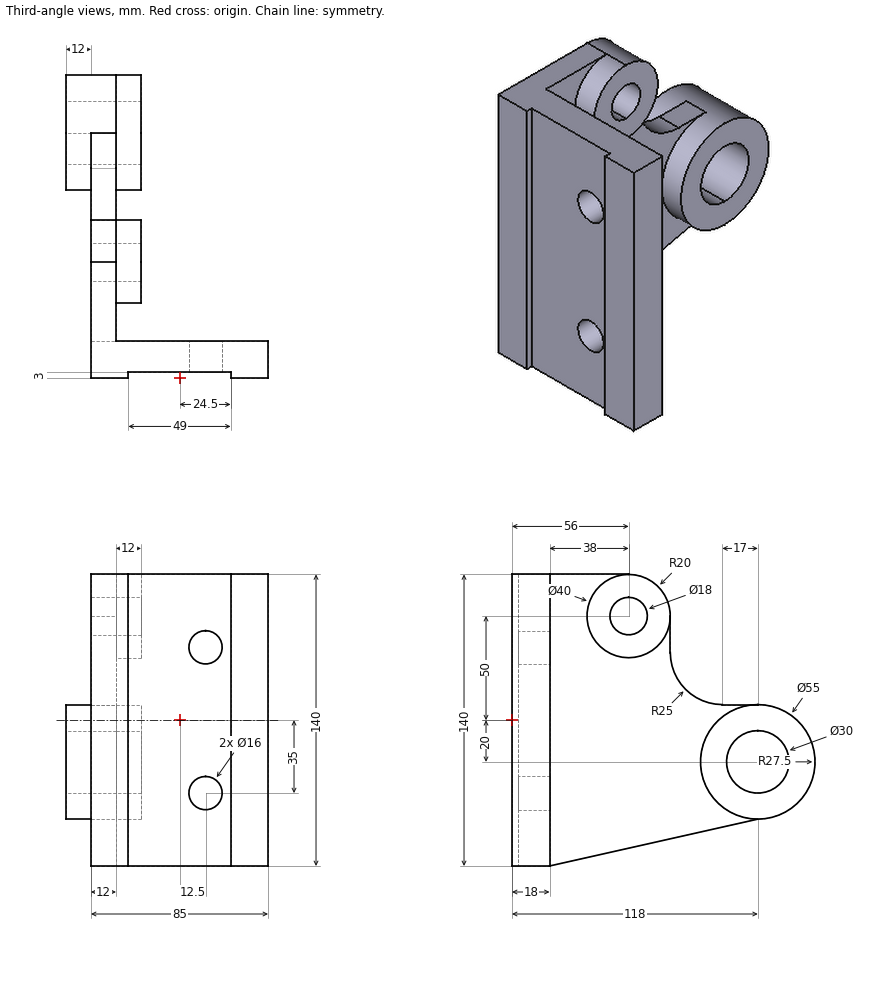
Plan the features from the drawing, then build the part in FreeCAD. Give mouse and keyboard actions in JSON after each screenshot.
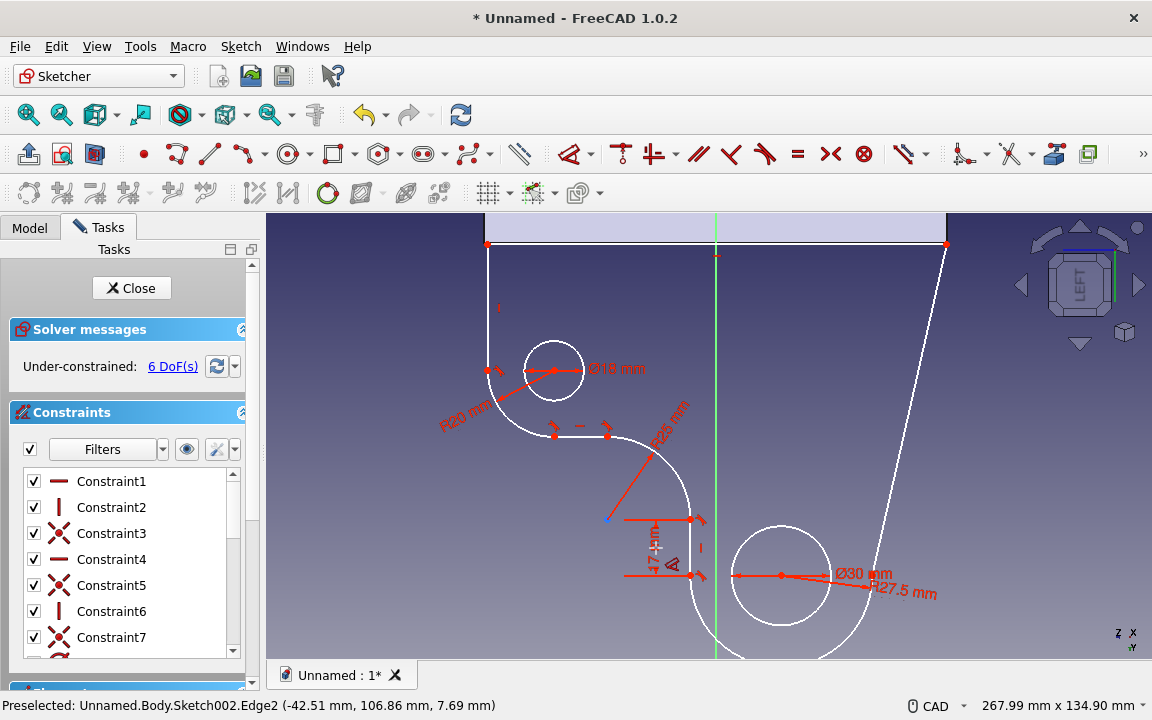
{"action": "left_click", "coordinate": [488, 282]}
{"action": "left_click", "coordinate": [454, 308]}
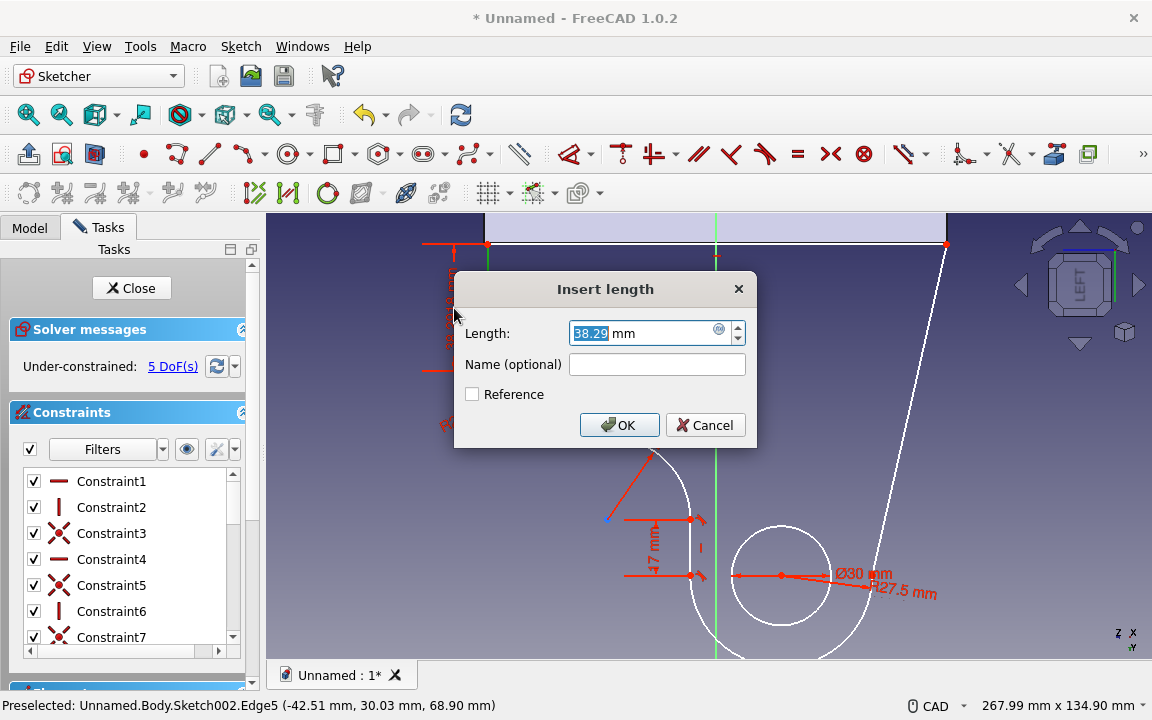
{"action": "type", "text": "38"}
{"action": "key", "text": "Return"}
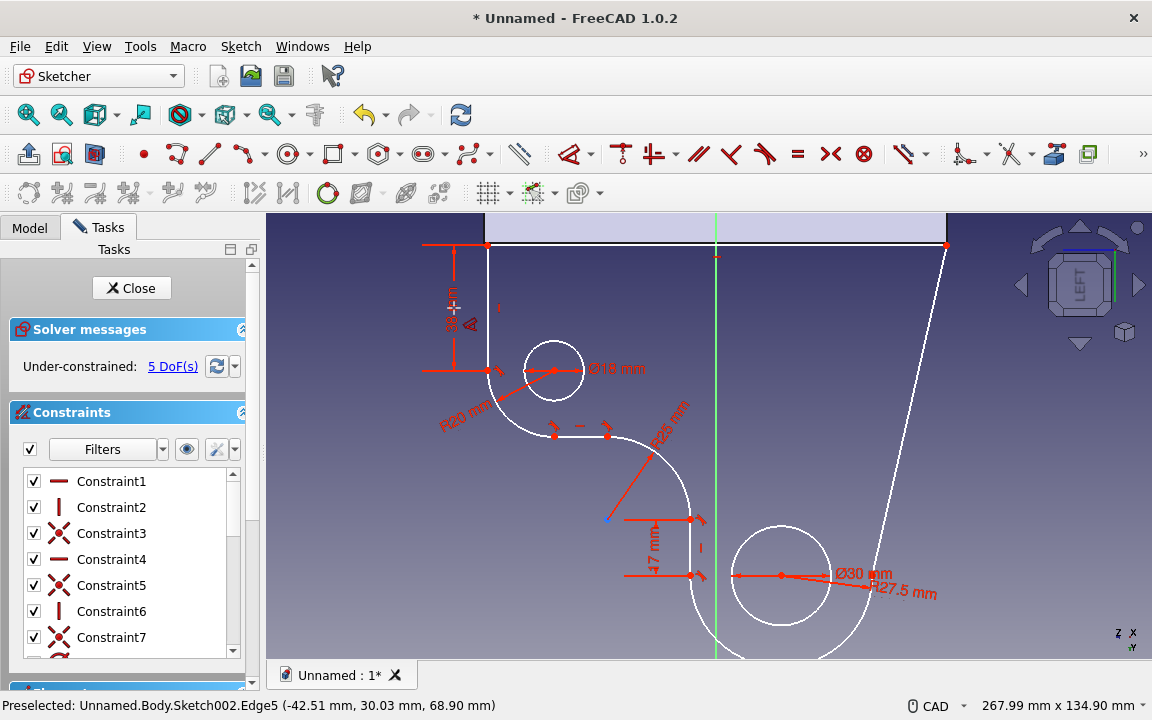
{"action": "left_click", "coordinate": [554, 371]}
{"action": "left_click", "coordinate": [635, 405]}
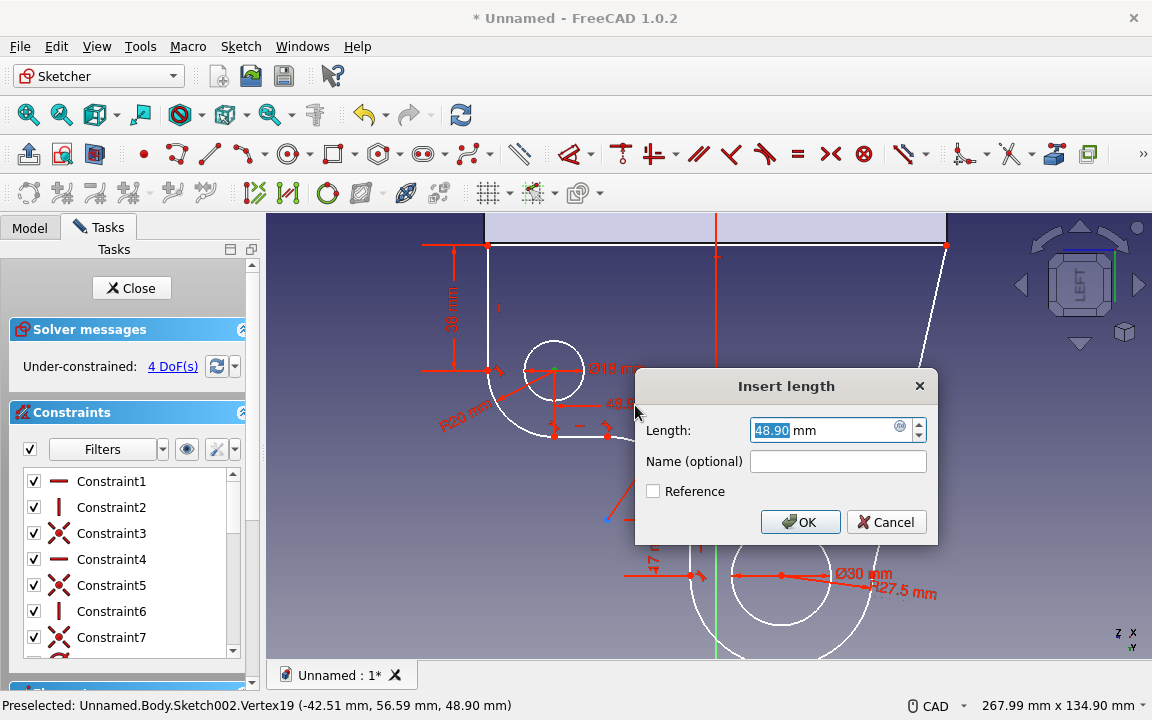
{"action": "type", "text": "50"}
{"action": "key", "text": "Return"}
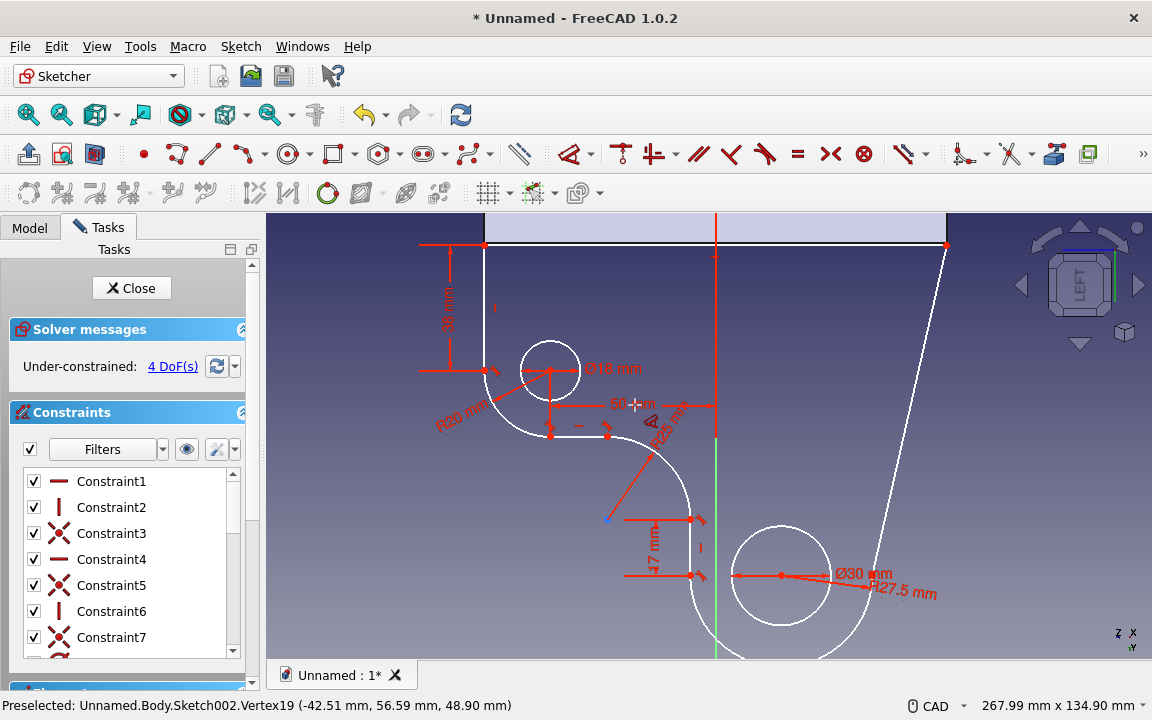
{"action": "left_click", "coordinate": [550, 371]}
{"action": "left_click", "coordinate": [516, 276]}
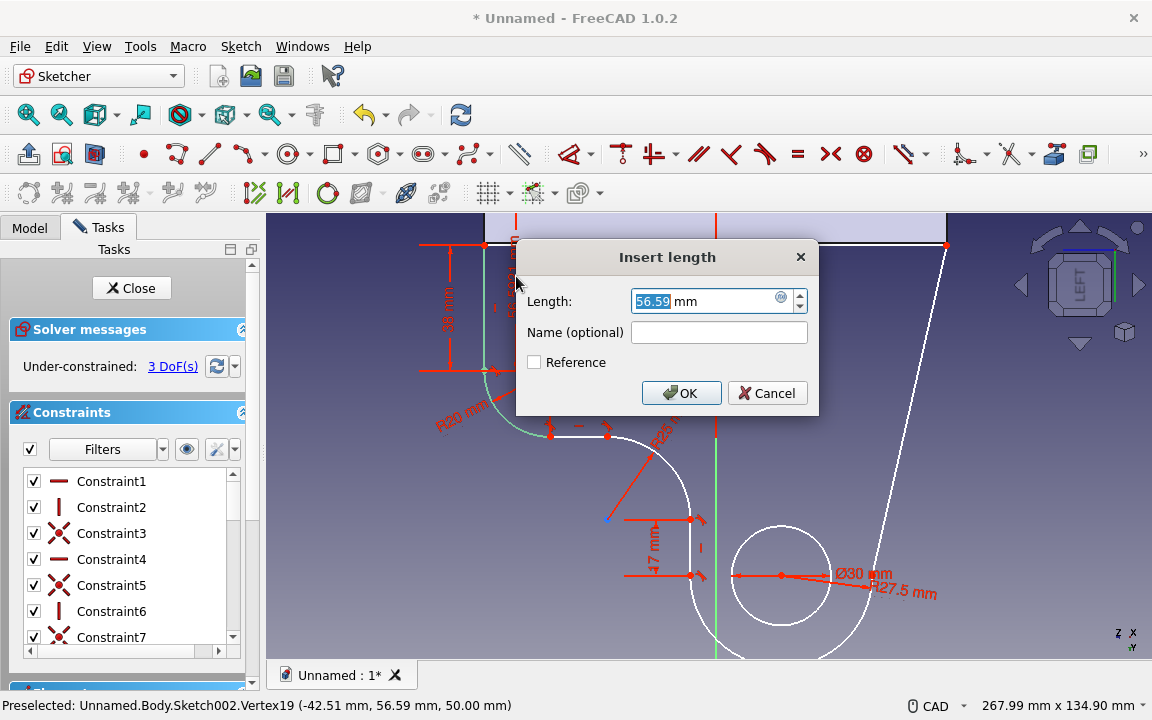
{"action": "type", "text": "56"}
{"action": "key", "text": "Return"}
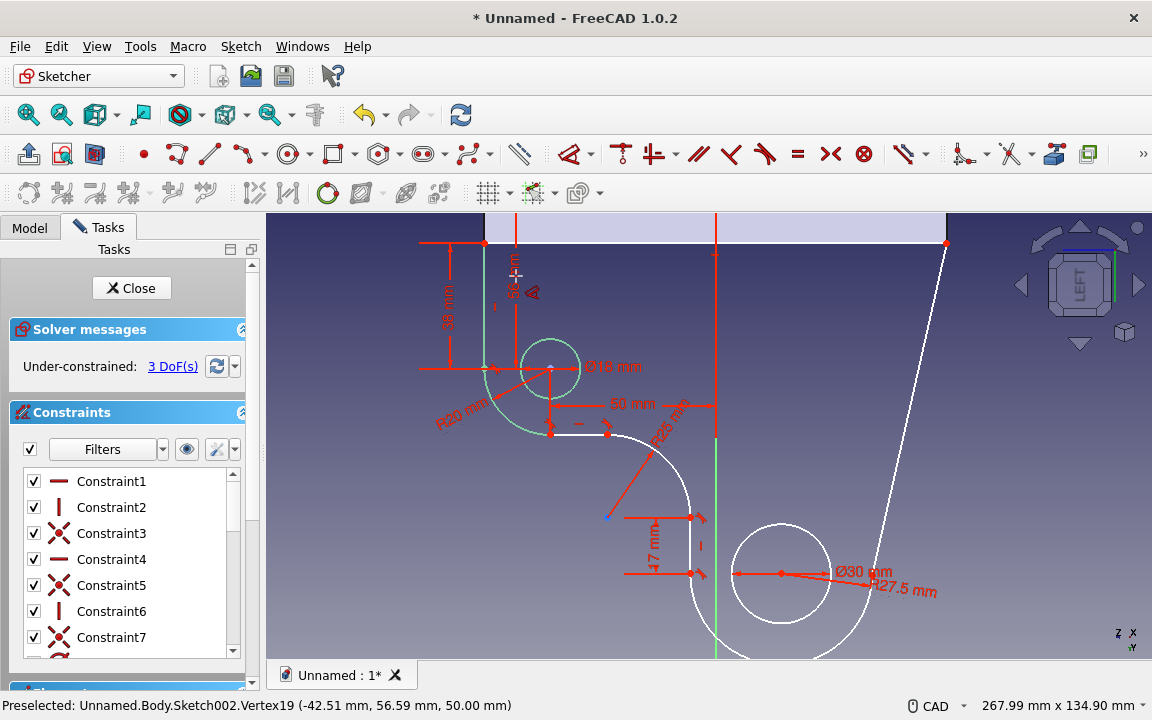
{"action": "left_click", "coordinate": [781, 574]}
{"action": "left_click", "coordinate": [771, 608]}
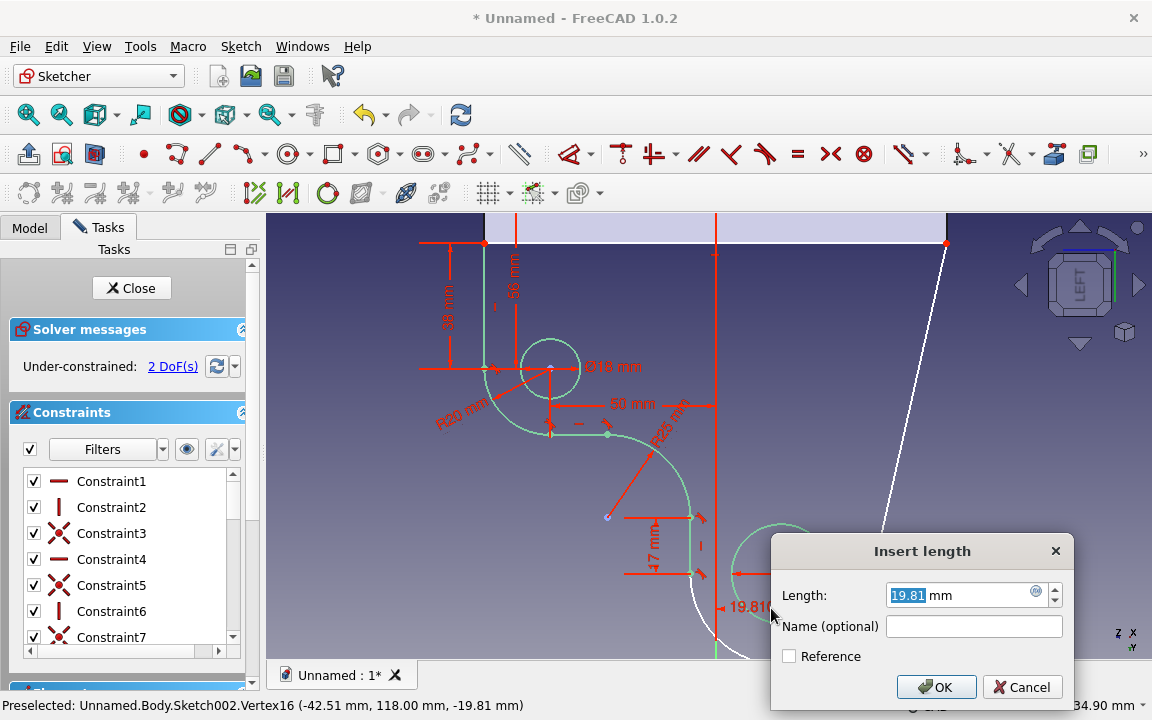
{"action": "type", "text": "20"}
{"action": "key", "text": "Return"}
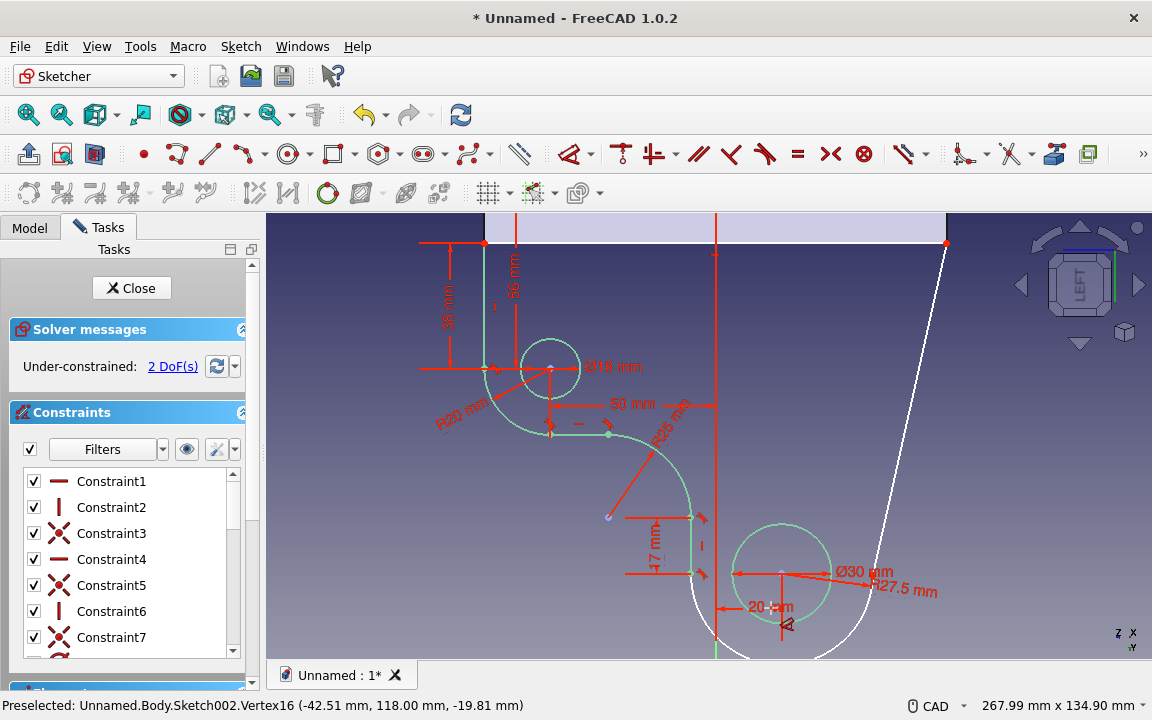
{"action": "left_click", "coordinate": [808, 243]}
{"action": "left_click", "coordinate": [609, 277]}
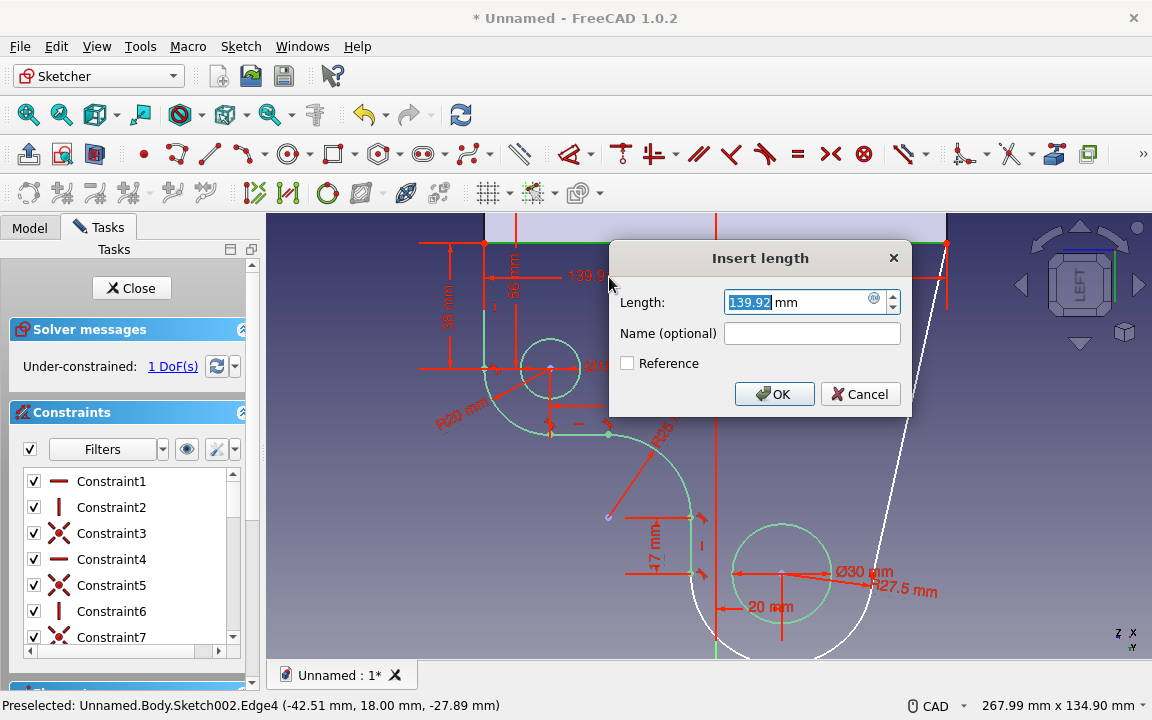
{"action": "type", "text": "140"}
{"action": "key", "text": "Return"}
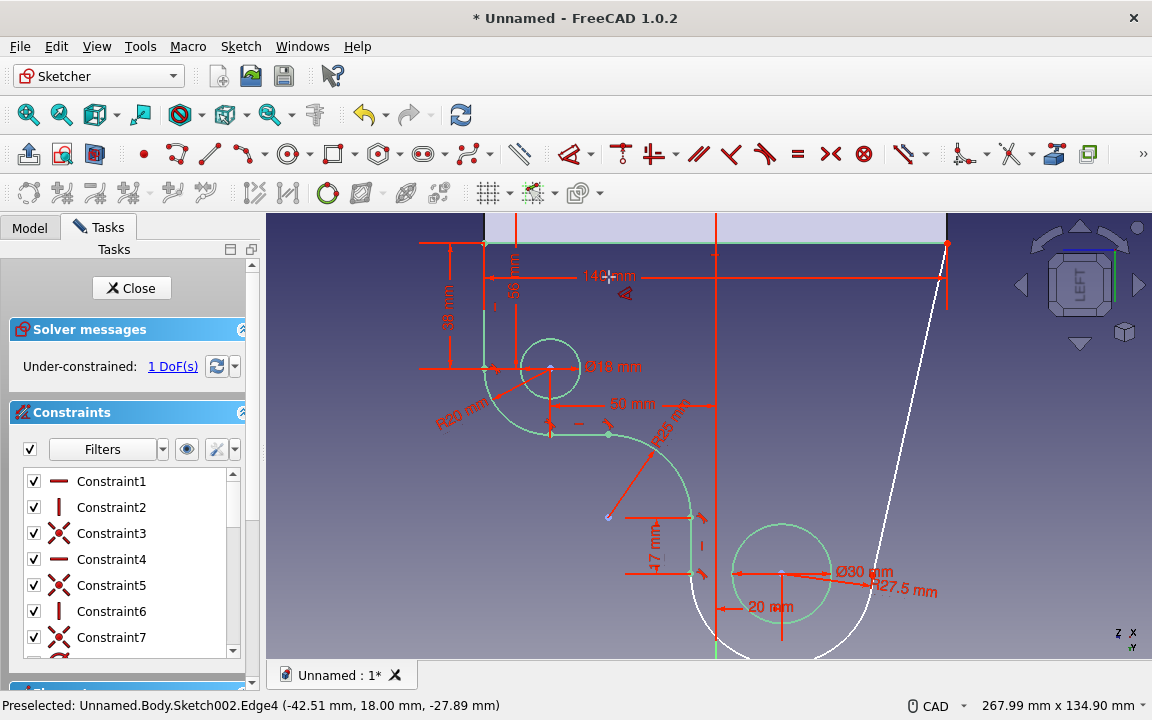
{"action": "left_click", "coordinate": [873, 575]}
{"action": "left_click", "coordinate": [907, 331]}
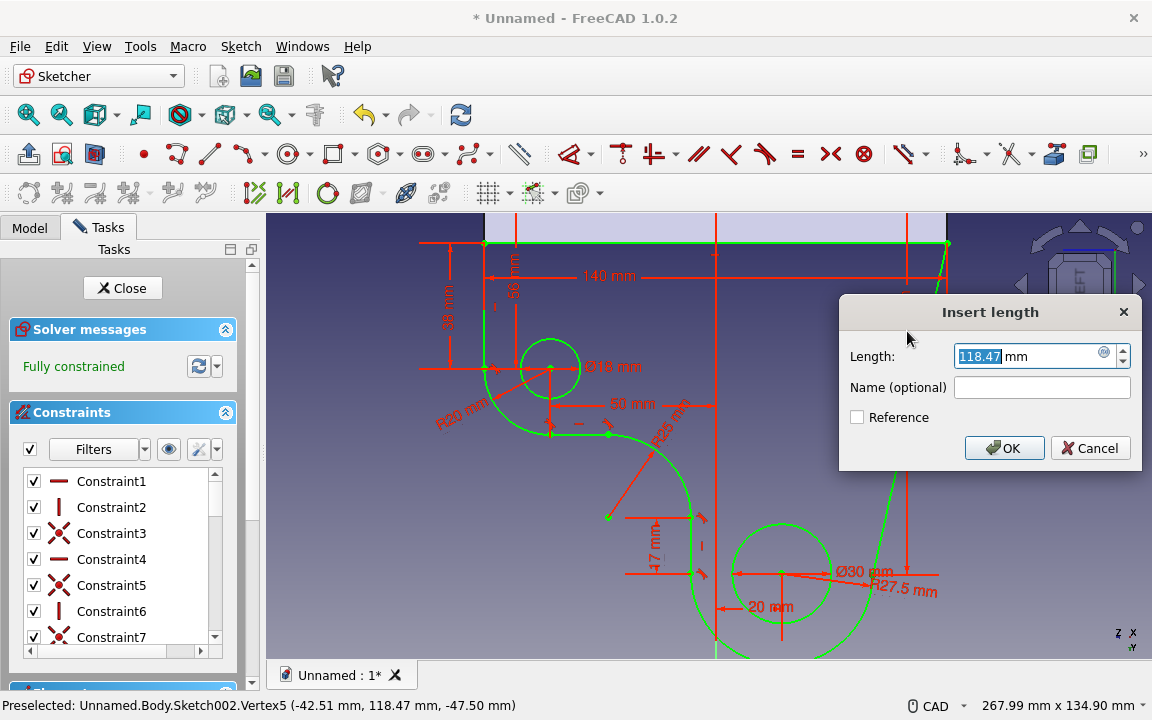
{"action": "type", "text": "118"}
{"action": "key", "text": "Return"}
{"action": "key", "text": "Escape"}